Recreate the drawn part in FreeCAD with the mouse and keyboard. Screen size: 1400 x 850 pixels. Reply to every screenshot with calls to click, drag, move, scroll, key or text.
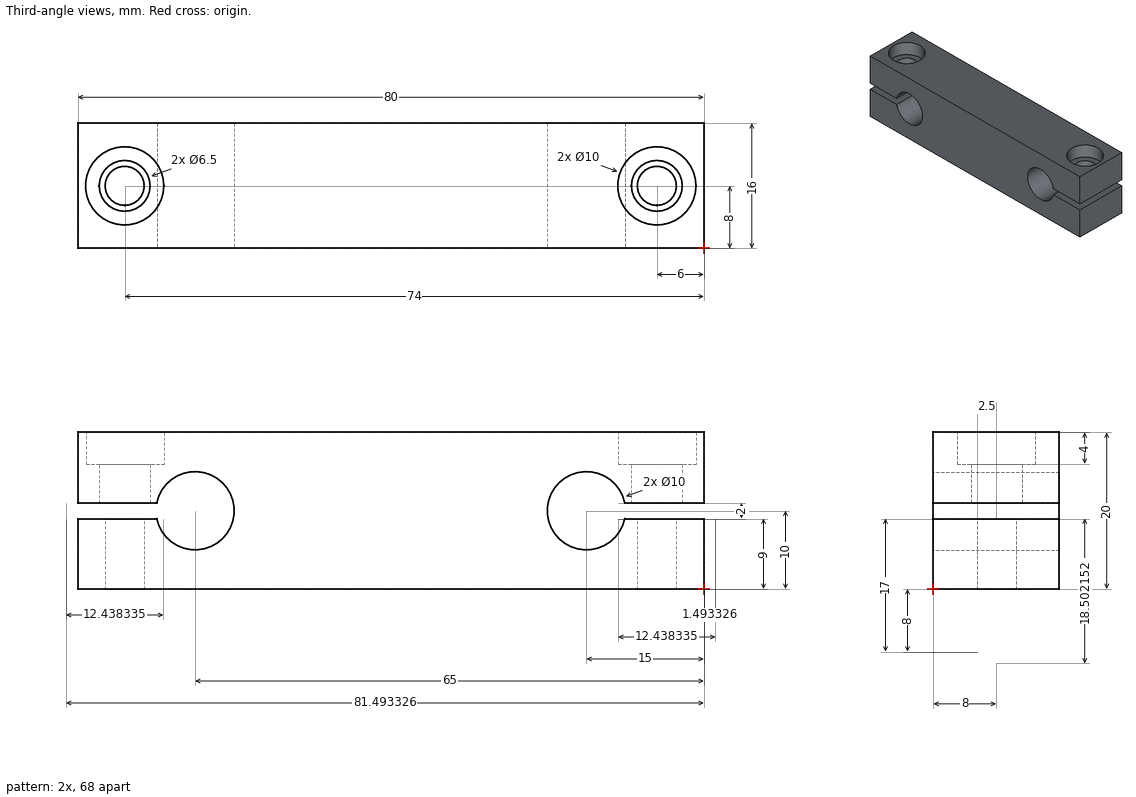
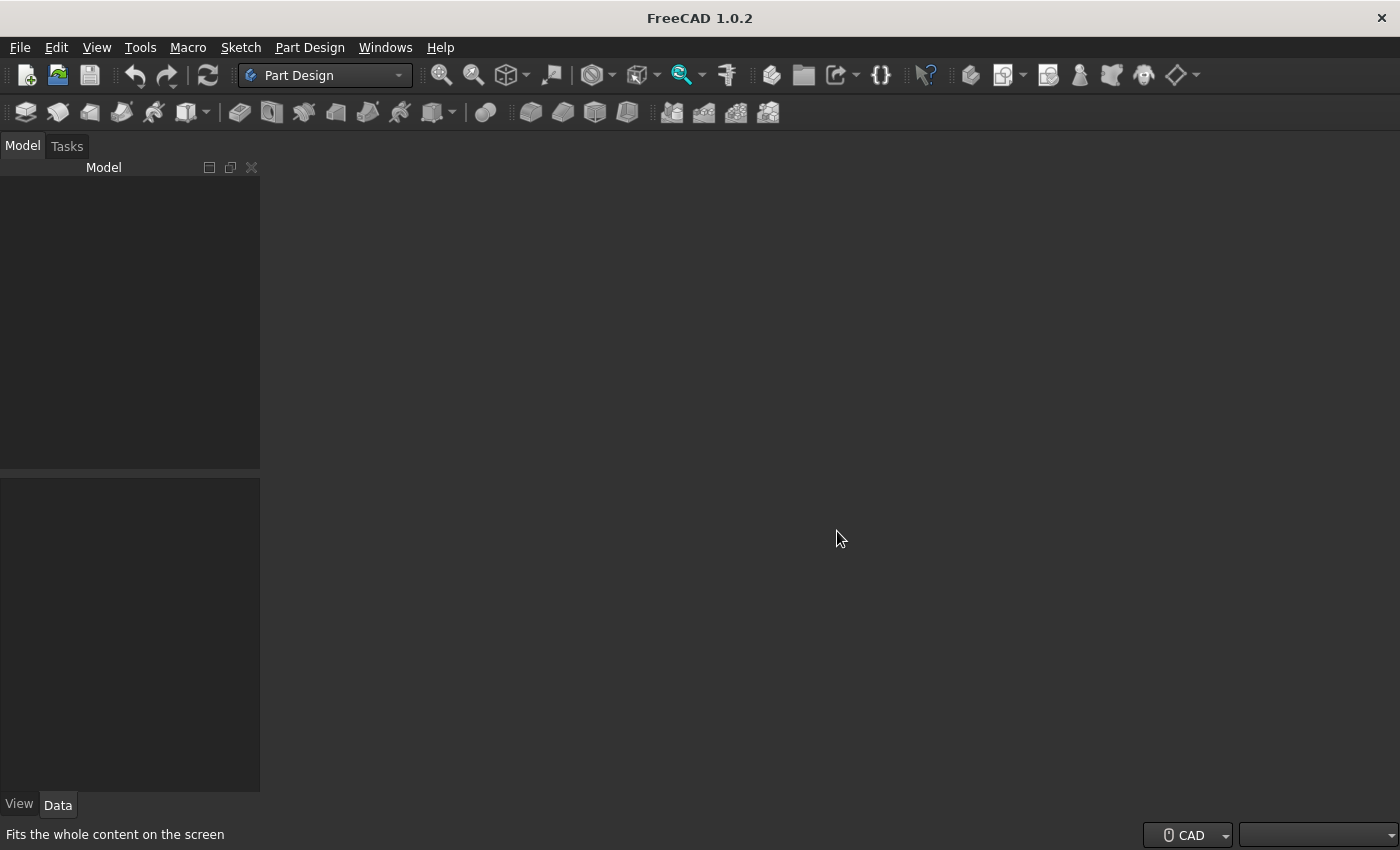
click(26, 76)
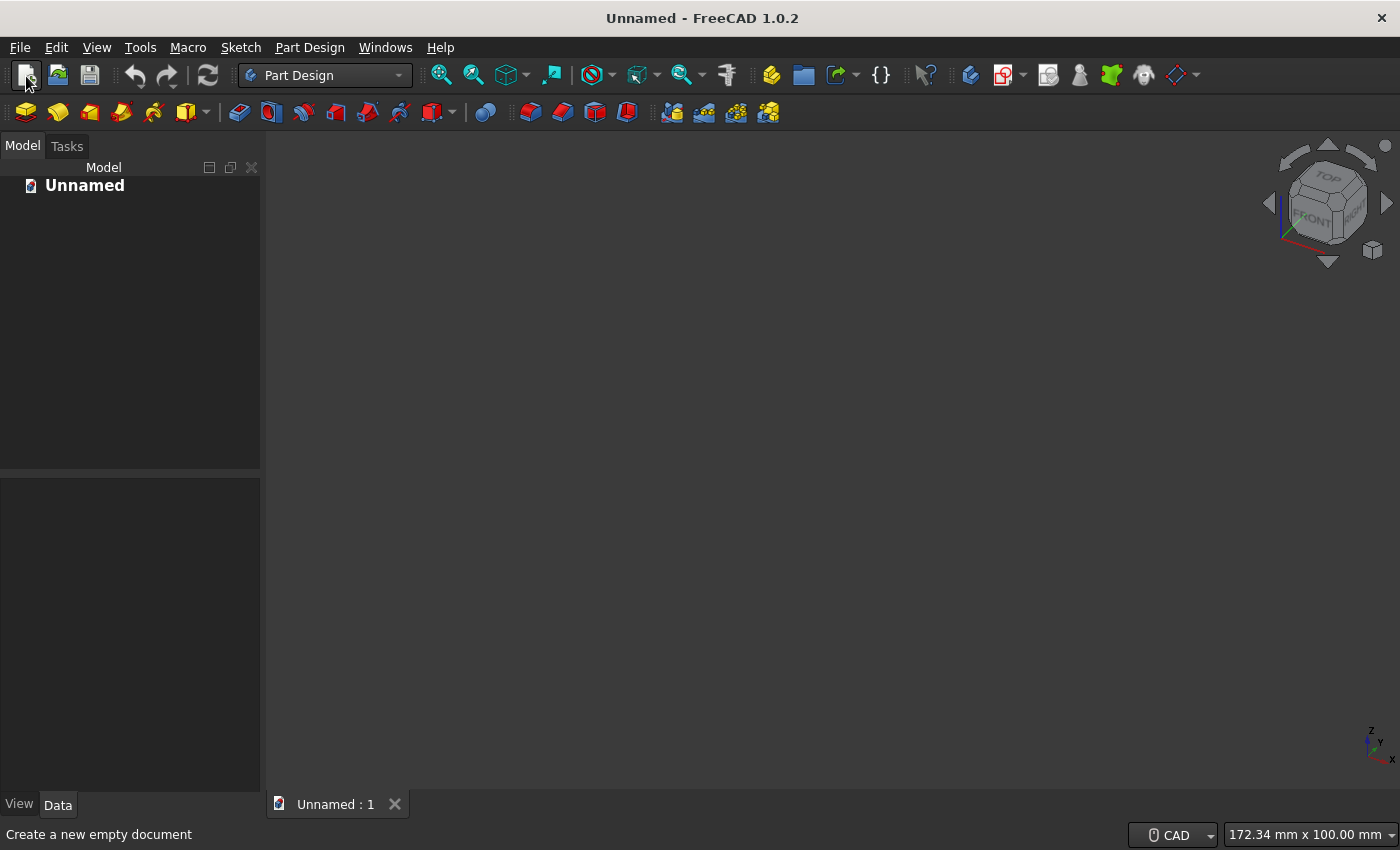
click(1004, 76)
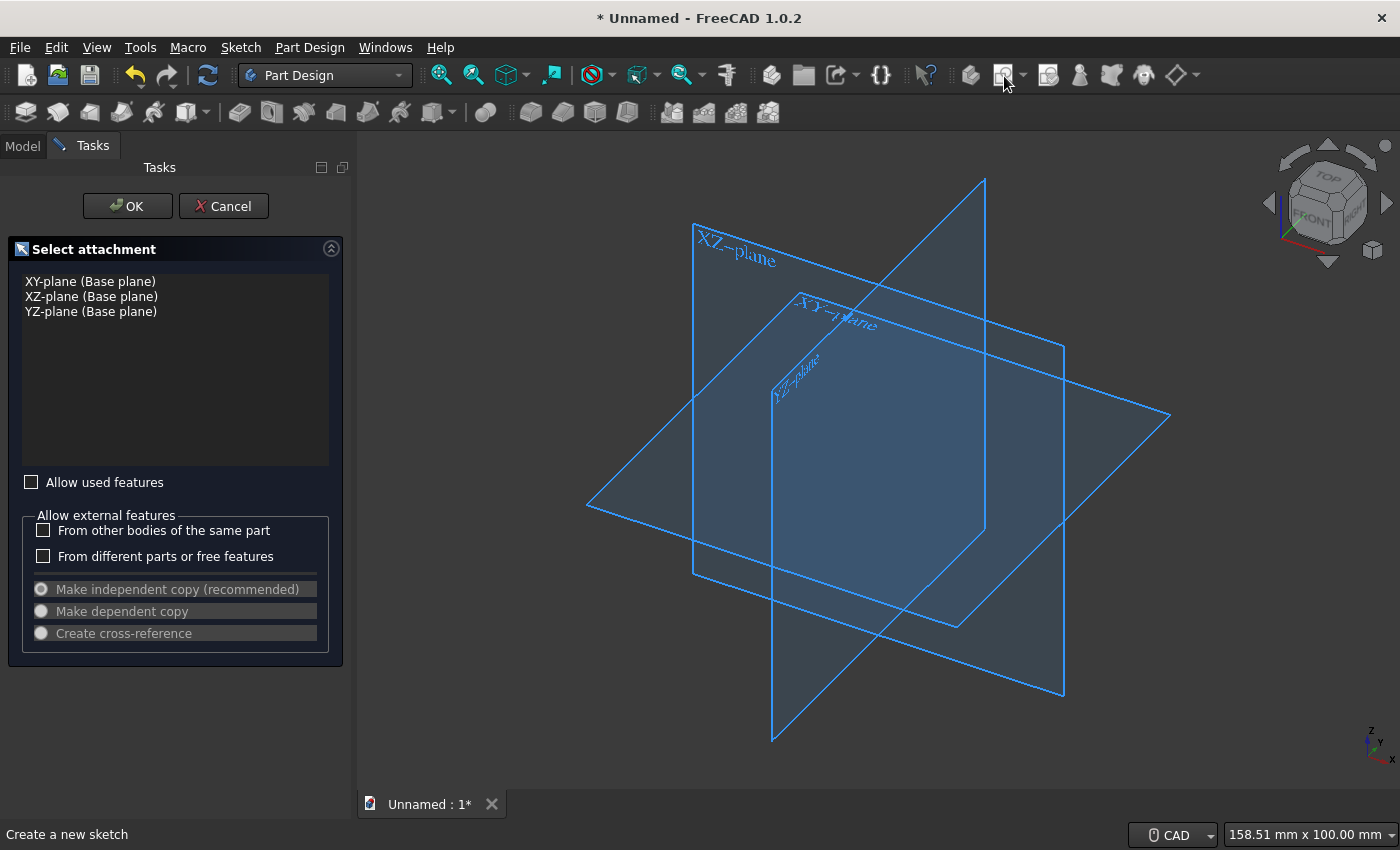
click(82, 282)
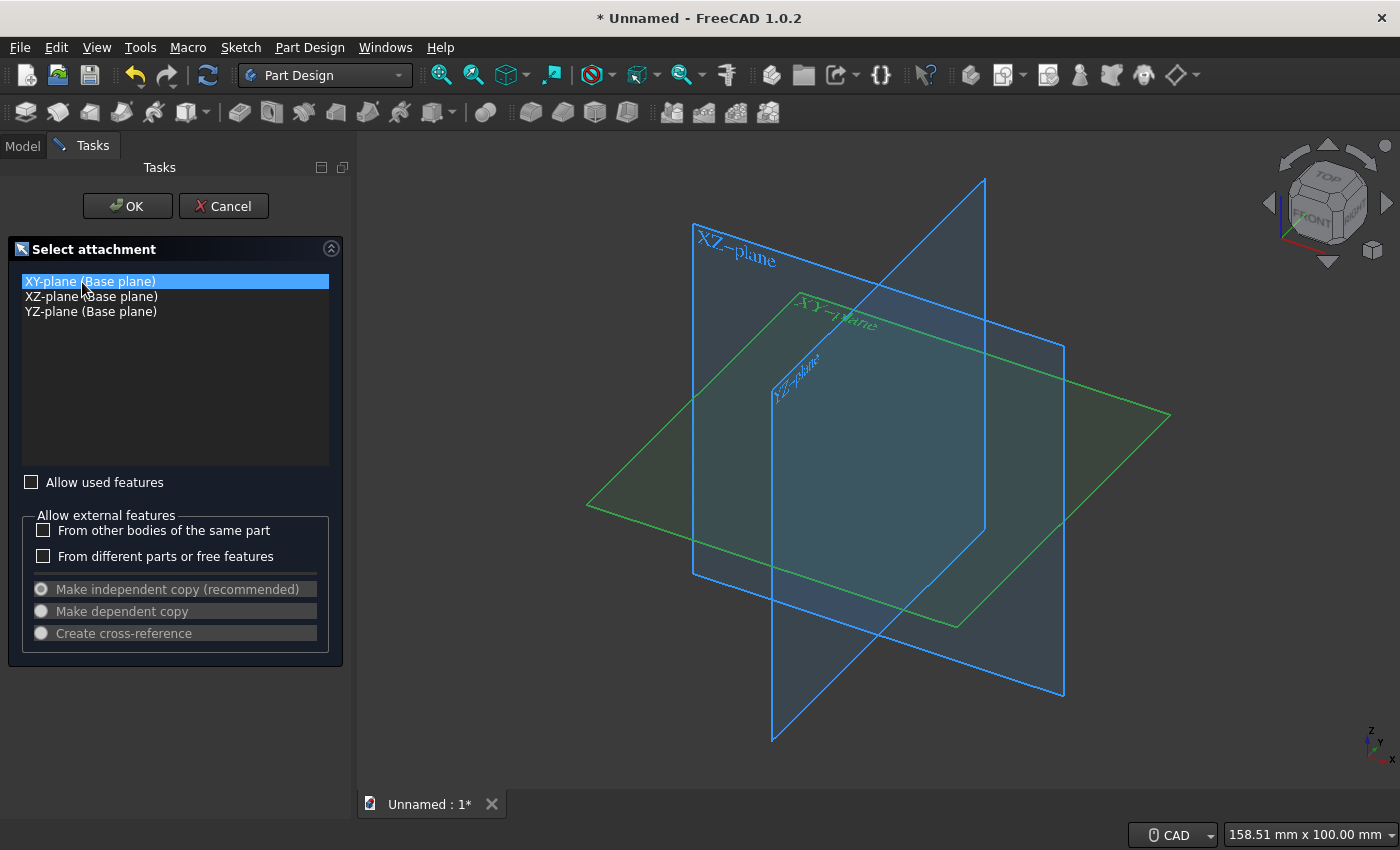
click(128, 206)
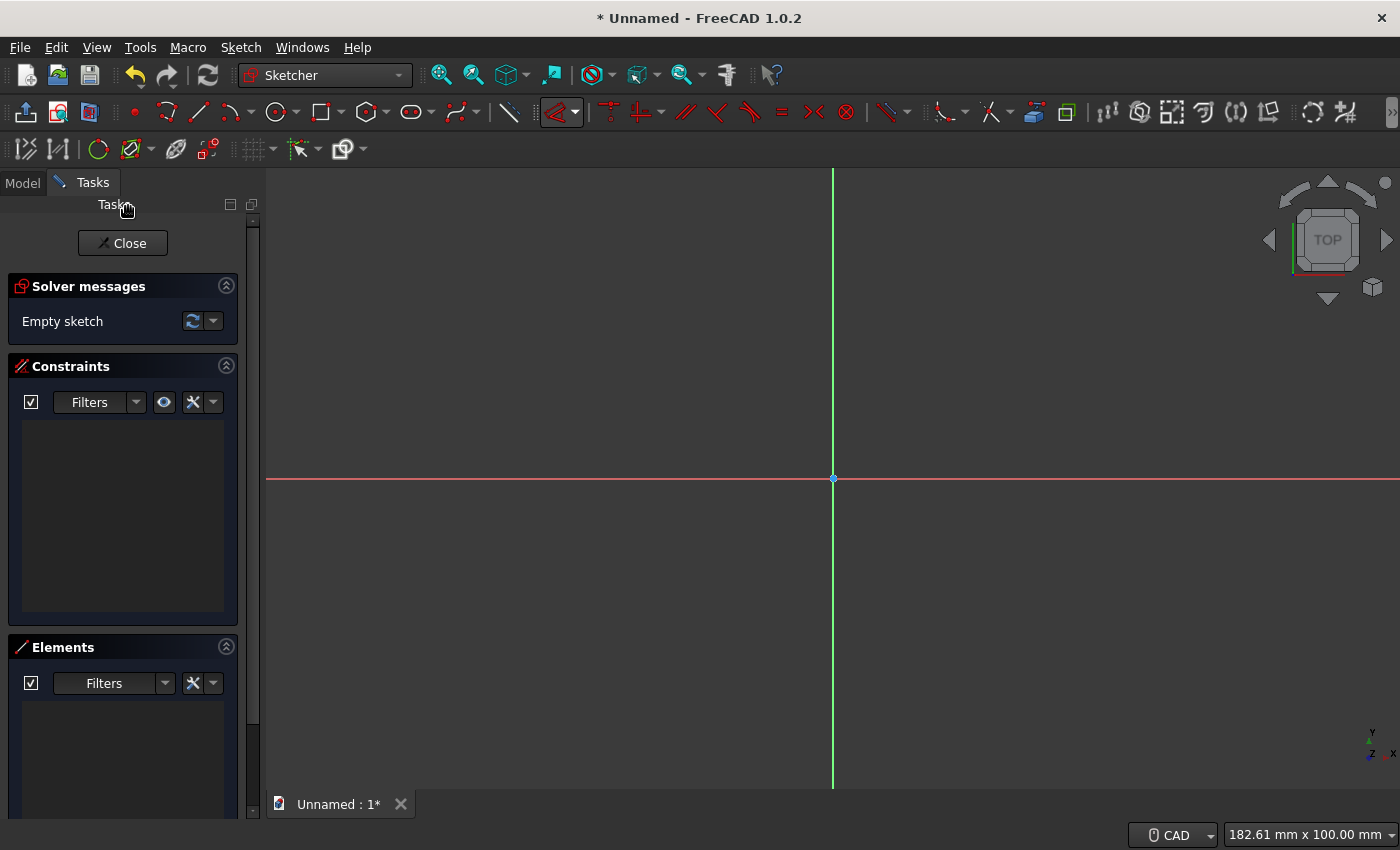
click(322, 112)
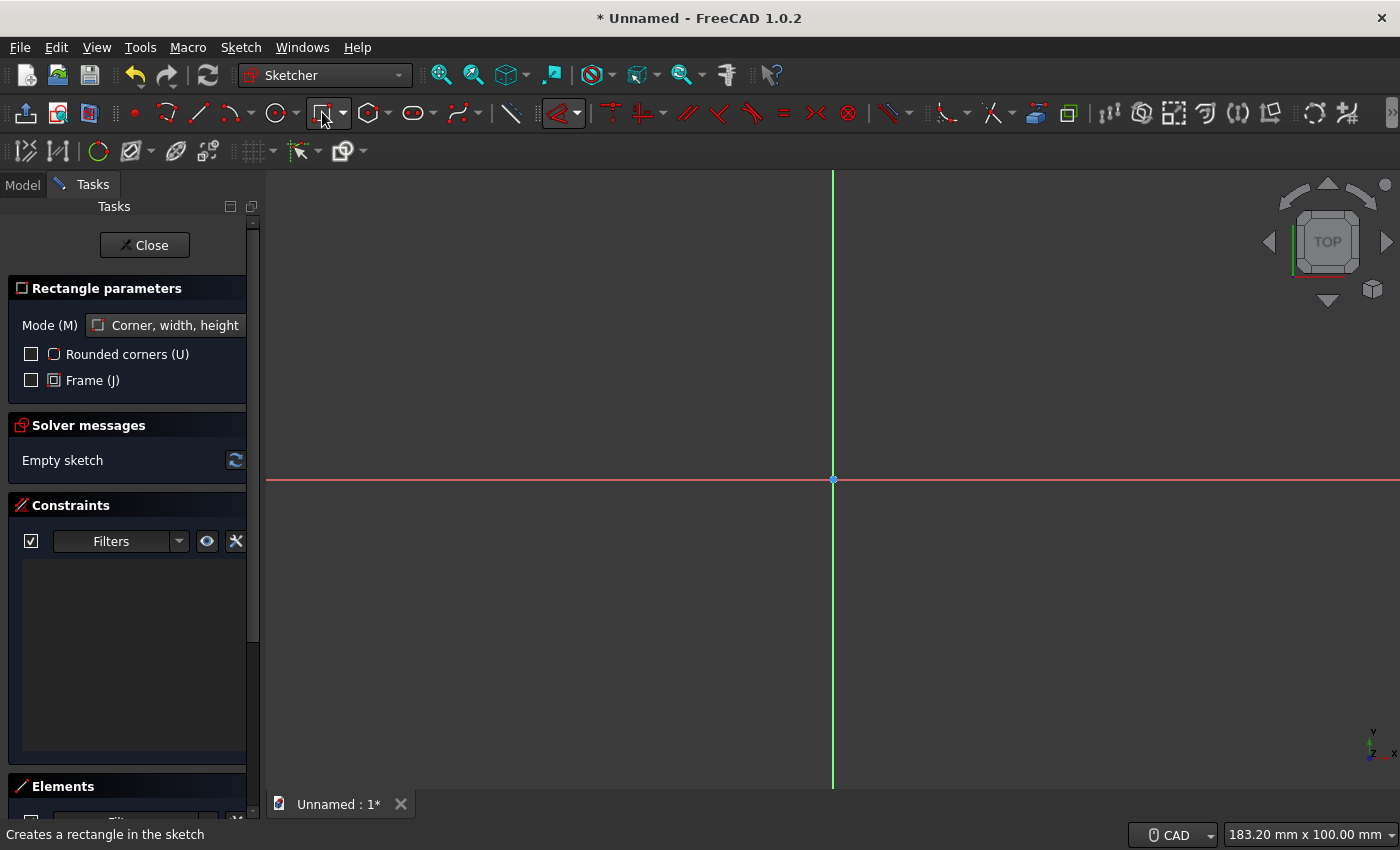
click(833, 480)
click(338, 380)
key(Escape)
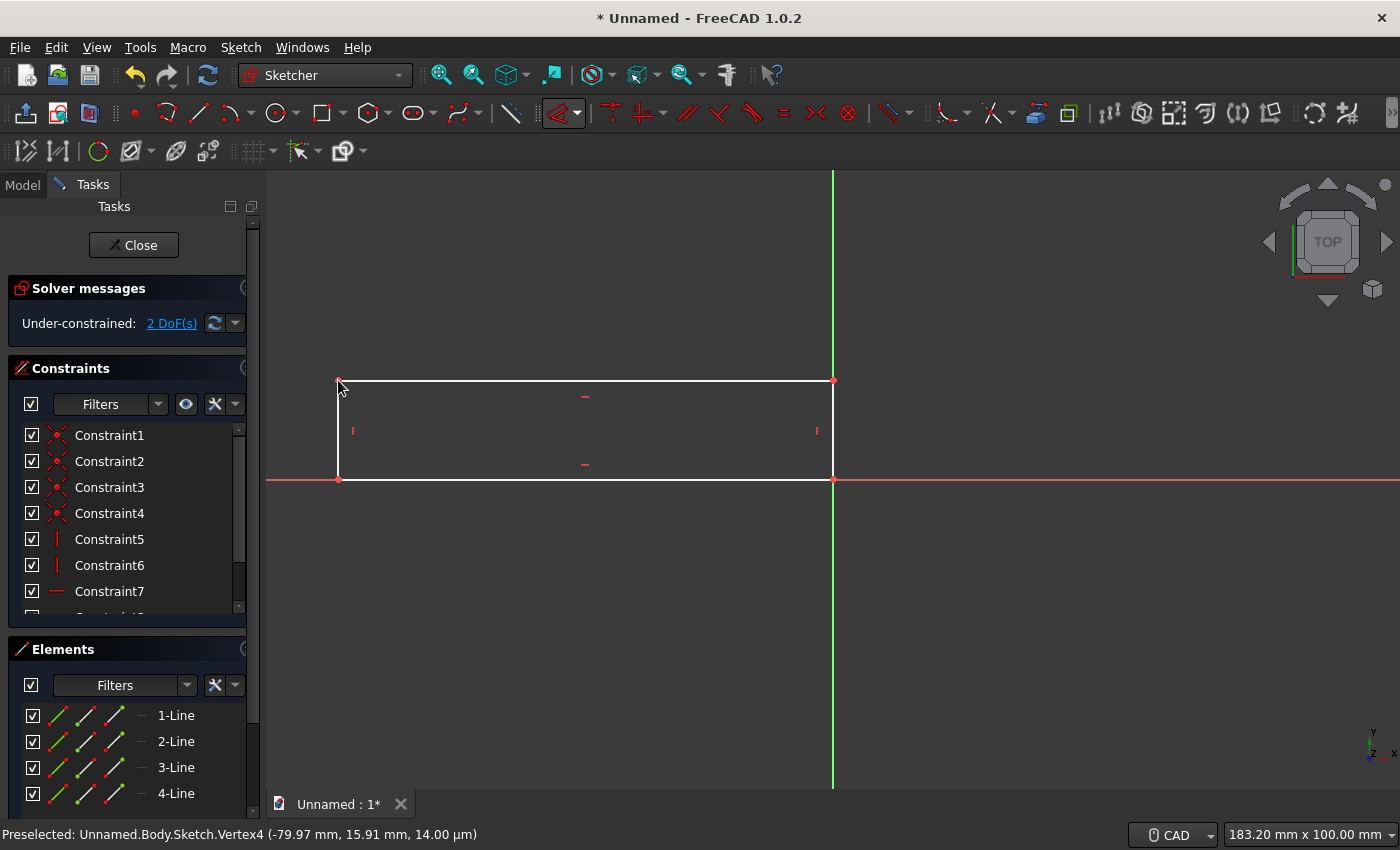
click(558, 114)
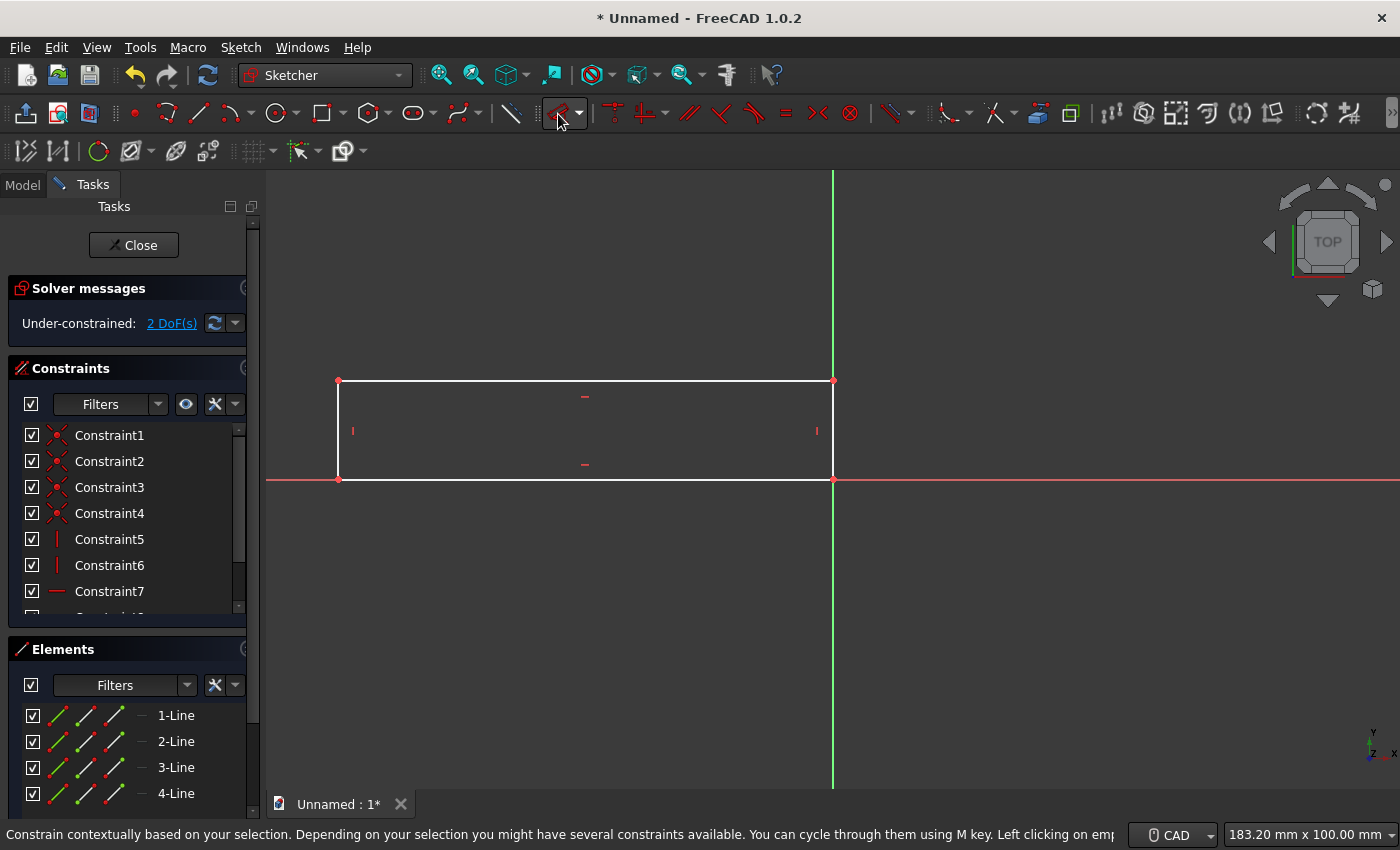
click(833, 450)
click(867, 430)